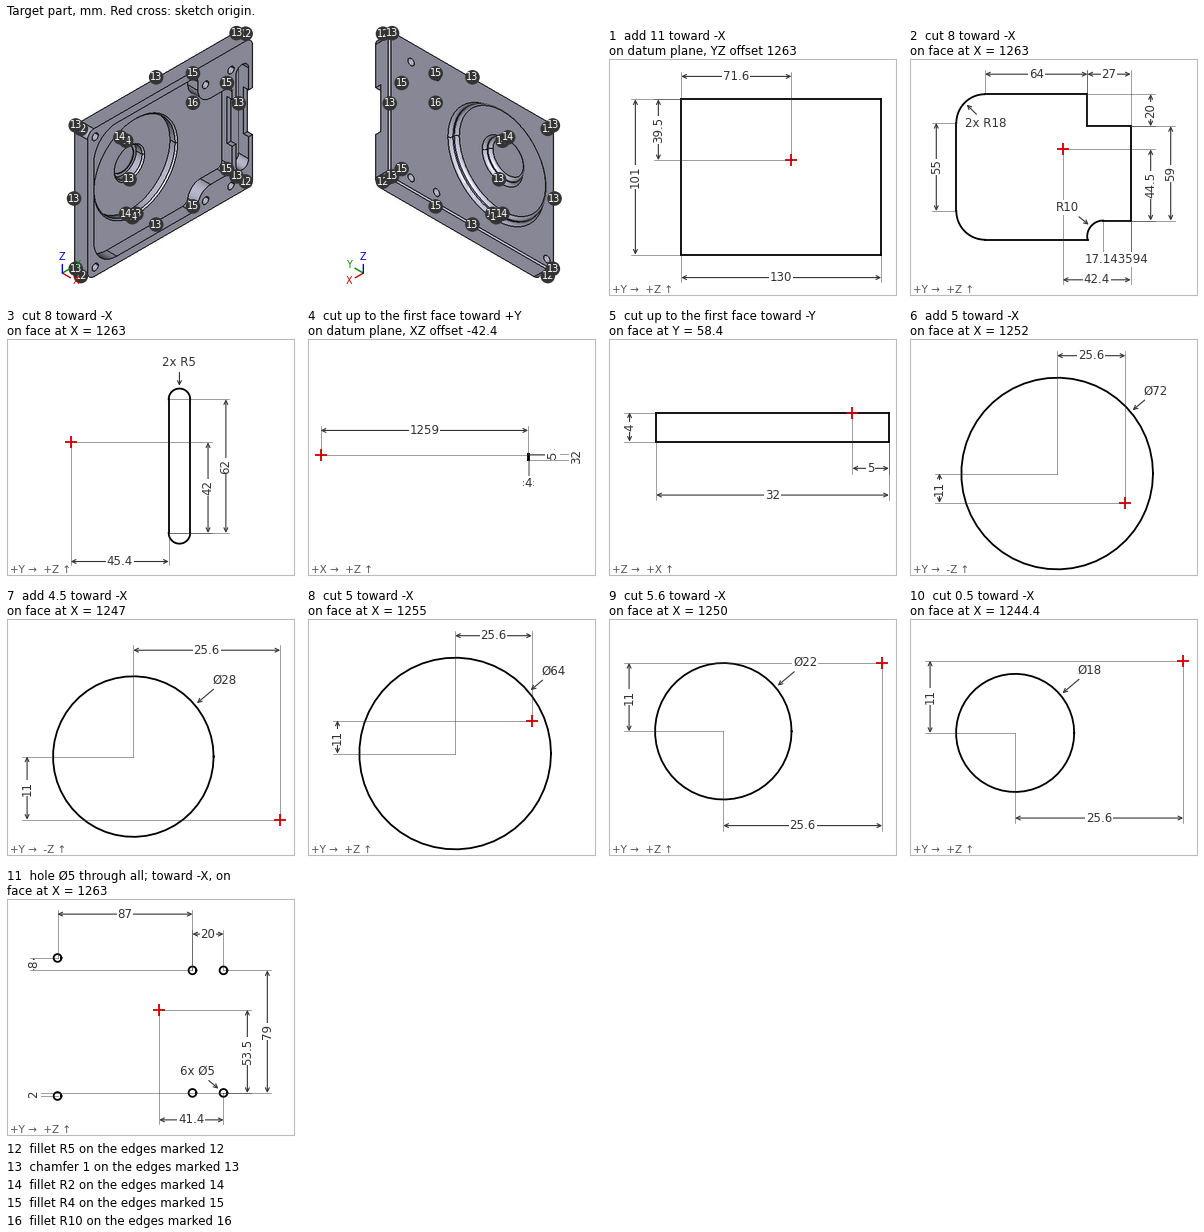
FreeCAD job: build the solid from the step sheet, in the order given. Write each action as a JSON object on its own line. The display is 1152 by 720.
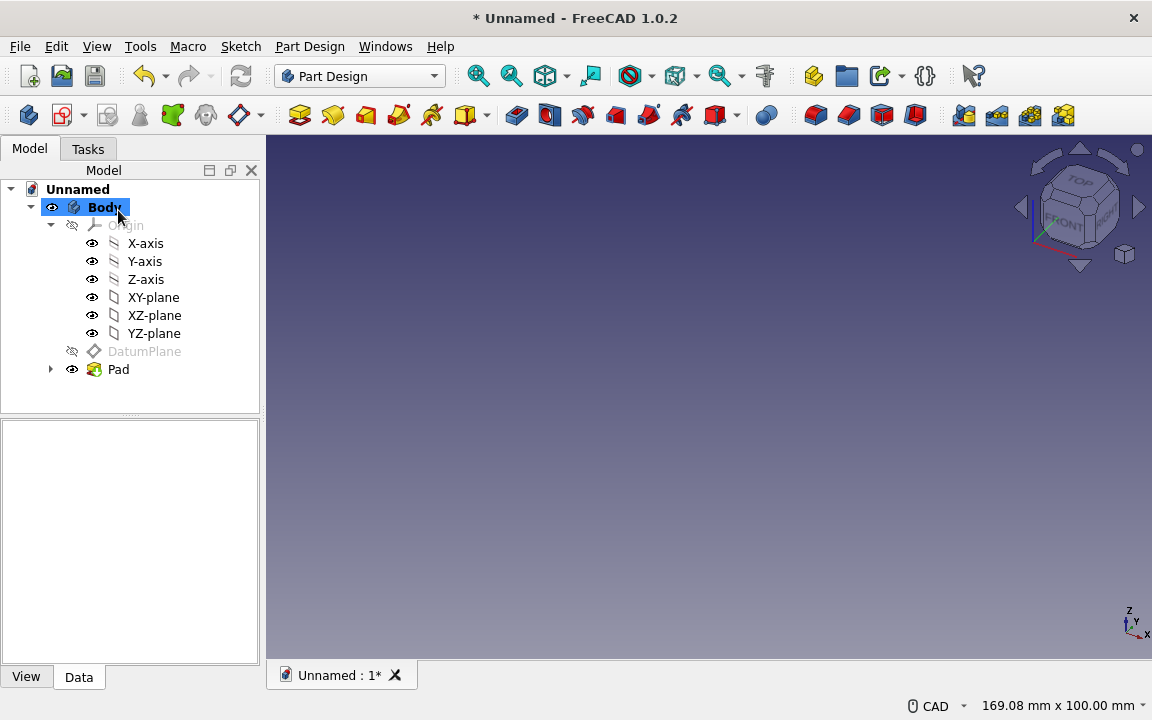
{"action": "left_click", "coordinate": [479, 76]}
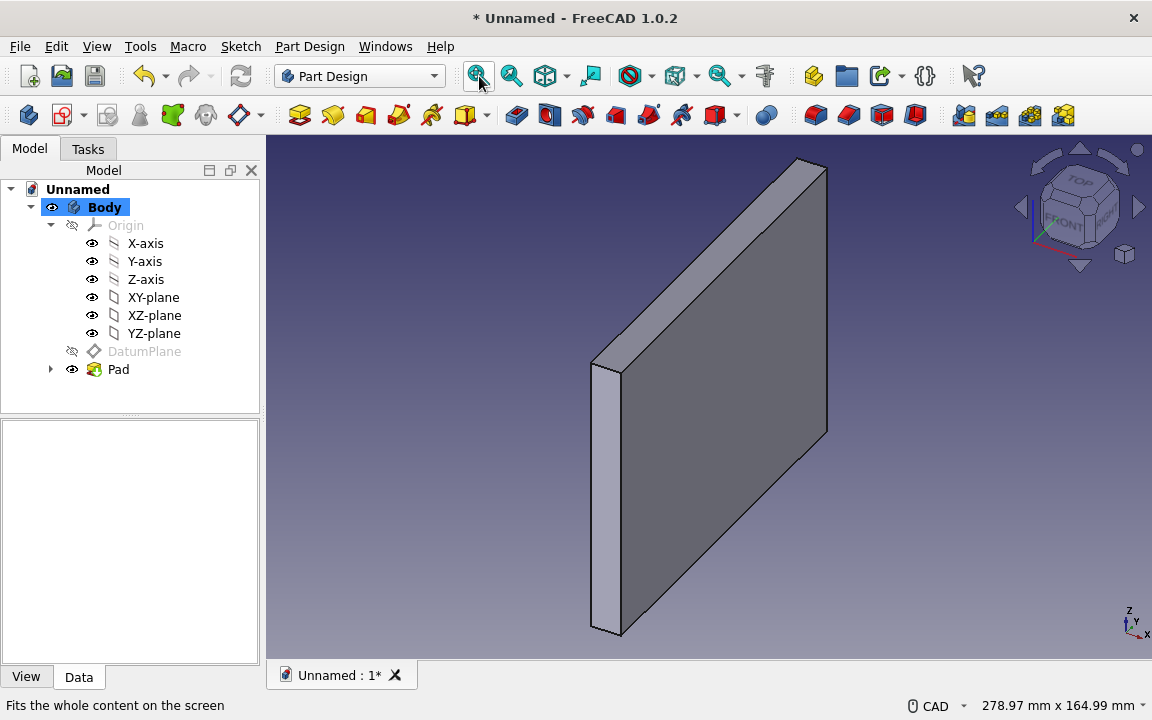
{"action": "left_click", "coordinate": [724, 401]}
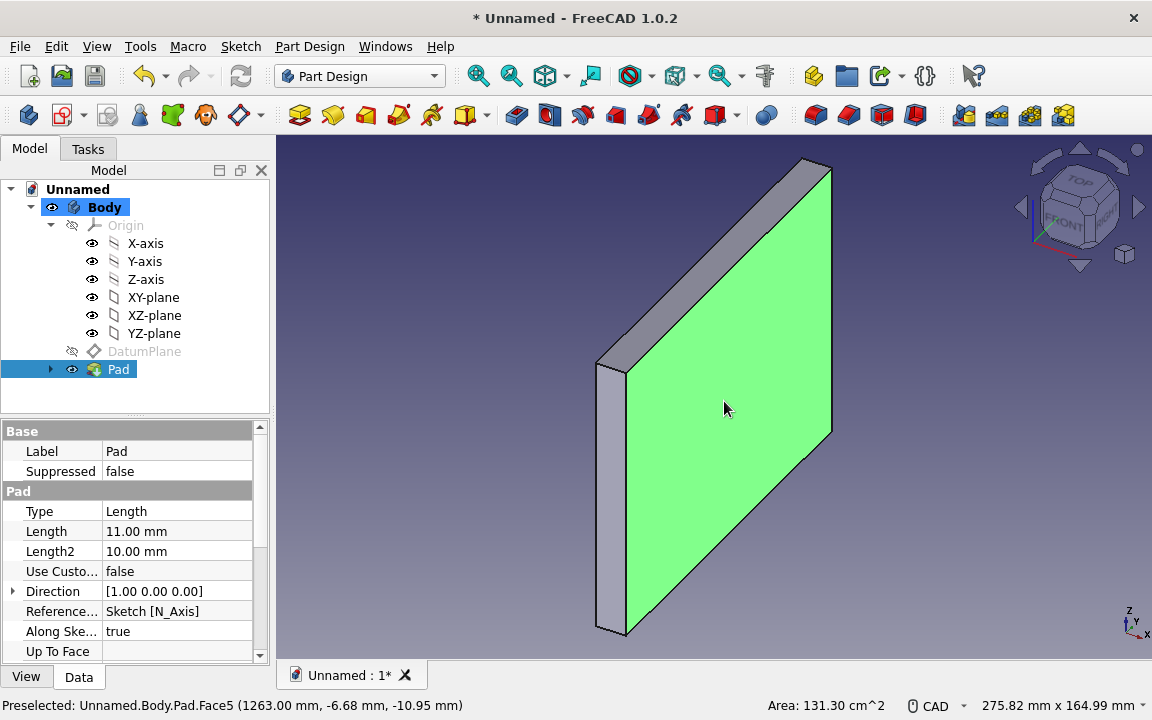
{"action": "left_click", "coordinate": [62, 116]}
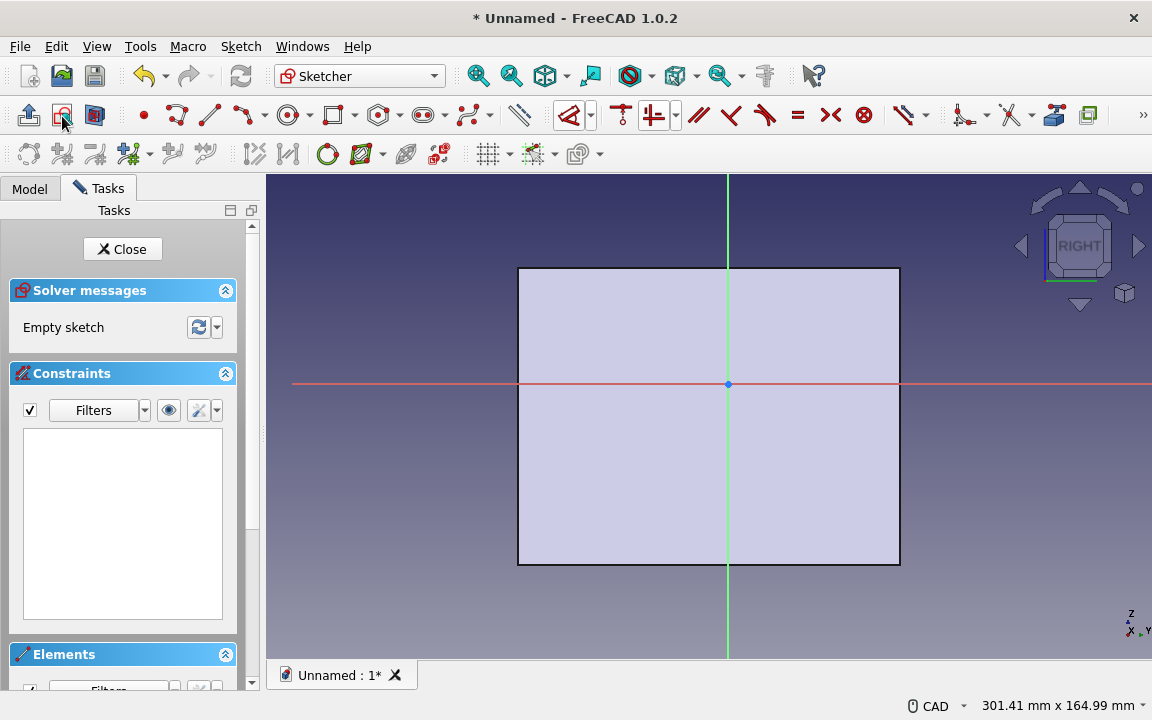
{"action": "left_click", "coordinate": [177, 116]}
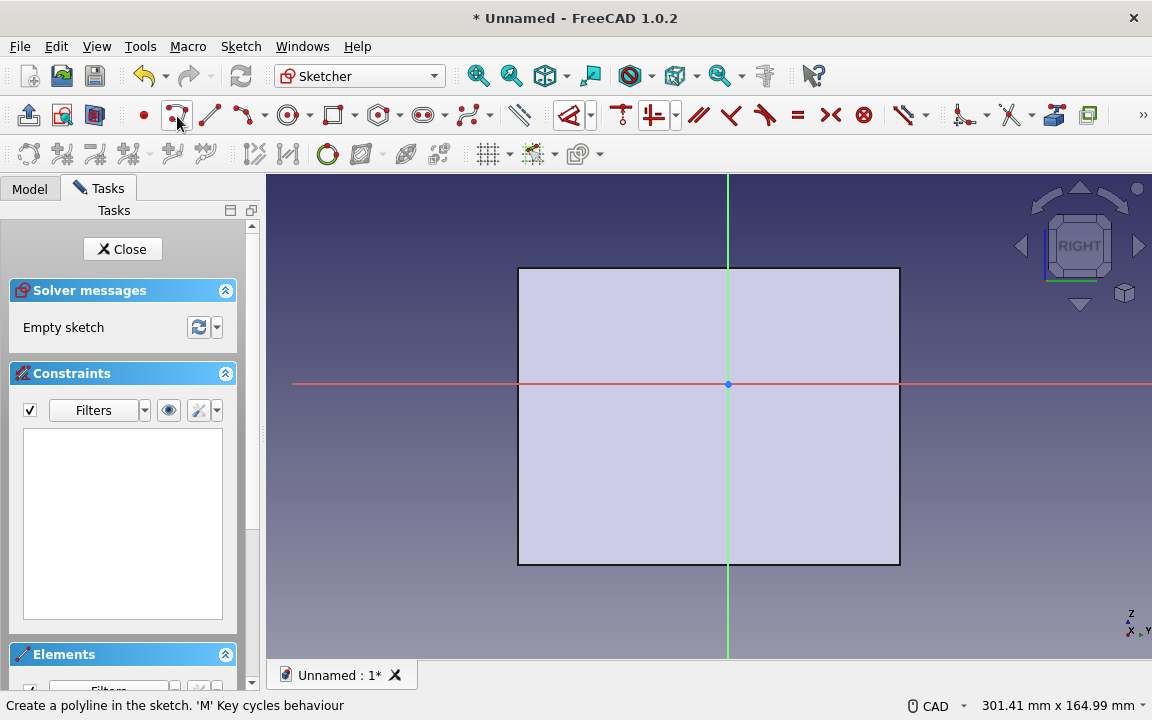
{"action": "left_click", "coordinate": [803, 515]}
{"action": "left_click", "coordinate": [853, 515]}
{"action": "left_click", "coordinate": [853, 342]}
{"action": "left_click", "coordinate": [774, 342]}
{"action": "left_click", "coordinate": [774, 283]}
{"action": "left_click", "coordinate": [586, 283]}
{"action": "right_click", "coordinate": [586, 283]}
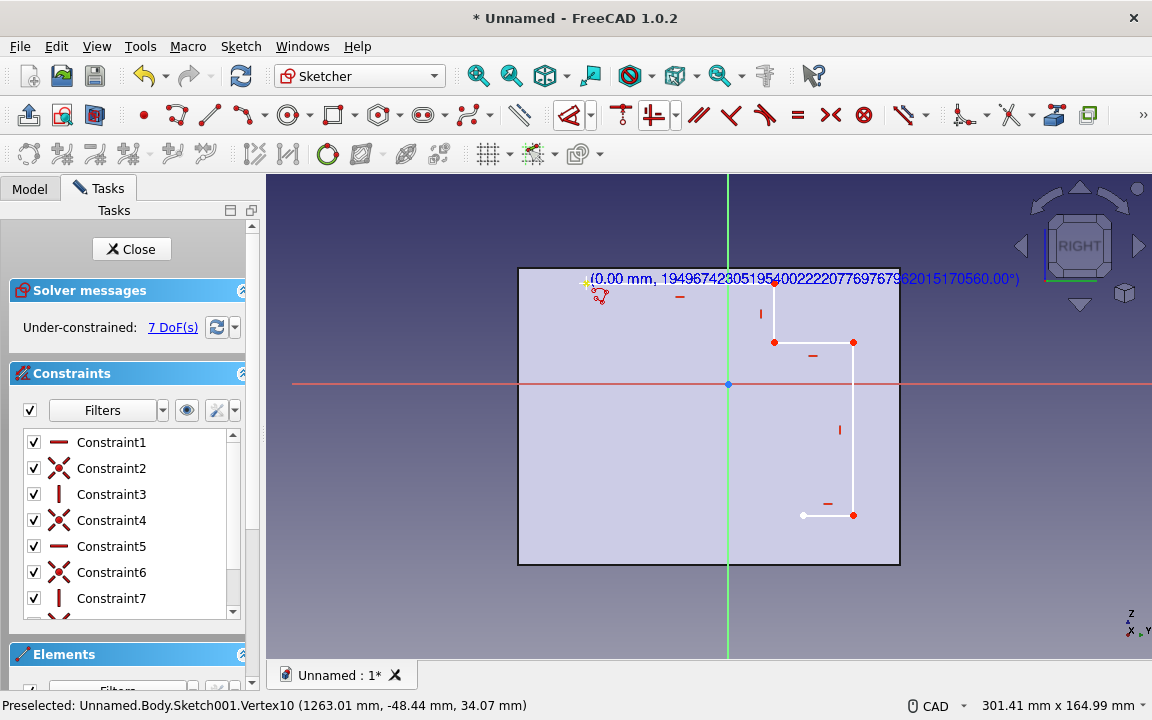
{"action": "left_click", "coordinate": [210, 116]}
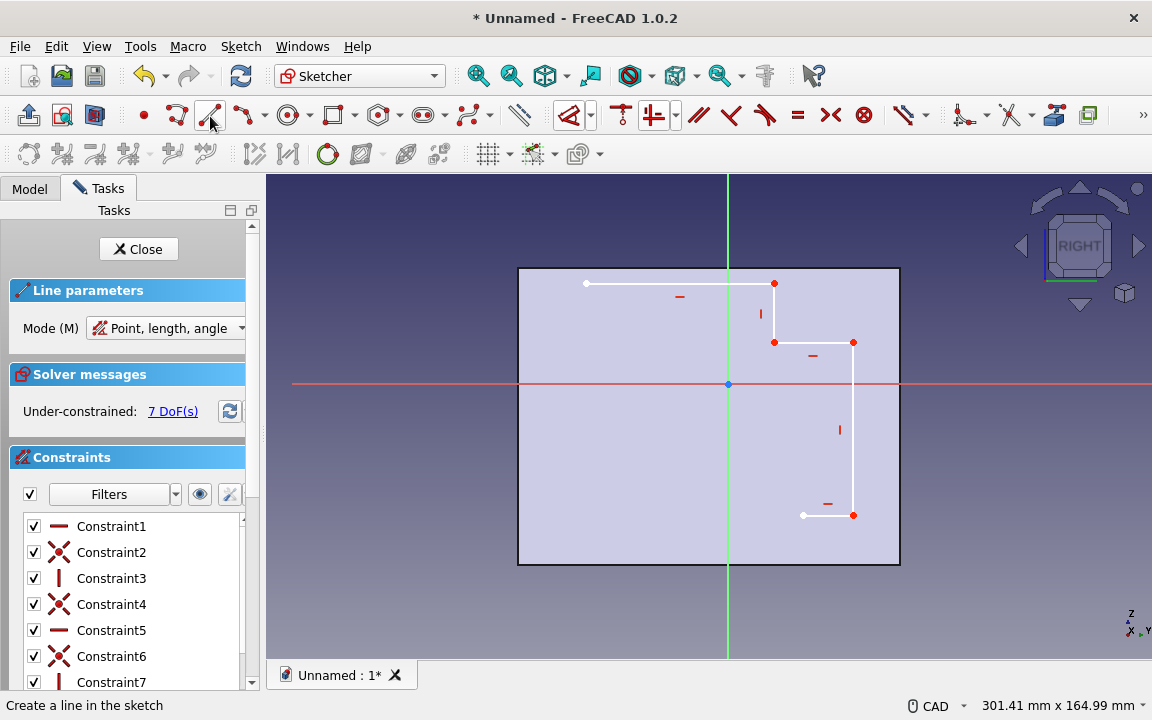
{"action": "left_click", "coordinate": [533, 336]}
{"action": "left_click", "coordinate": [533, 497]}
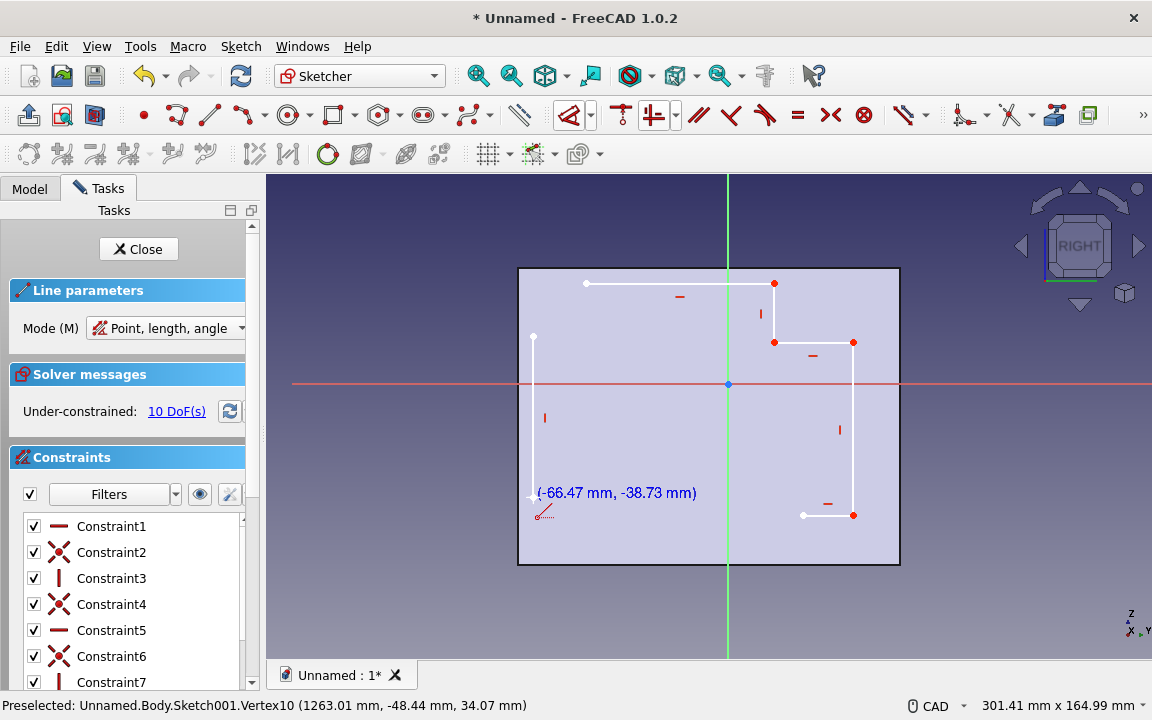
{"action": "left_click", "coordinate": [586, 550]}
{"action": "left_click", "coordinate": [774, 550]}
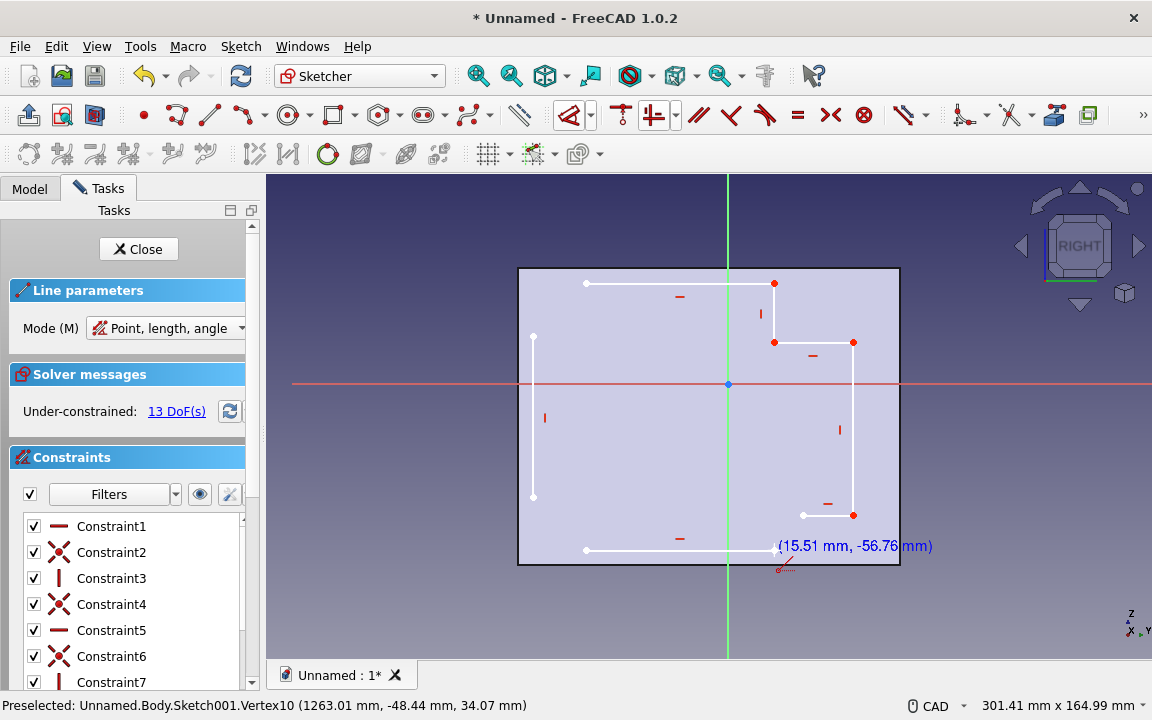
{"action": "left_click", "coordinate": [242, 116]}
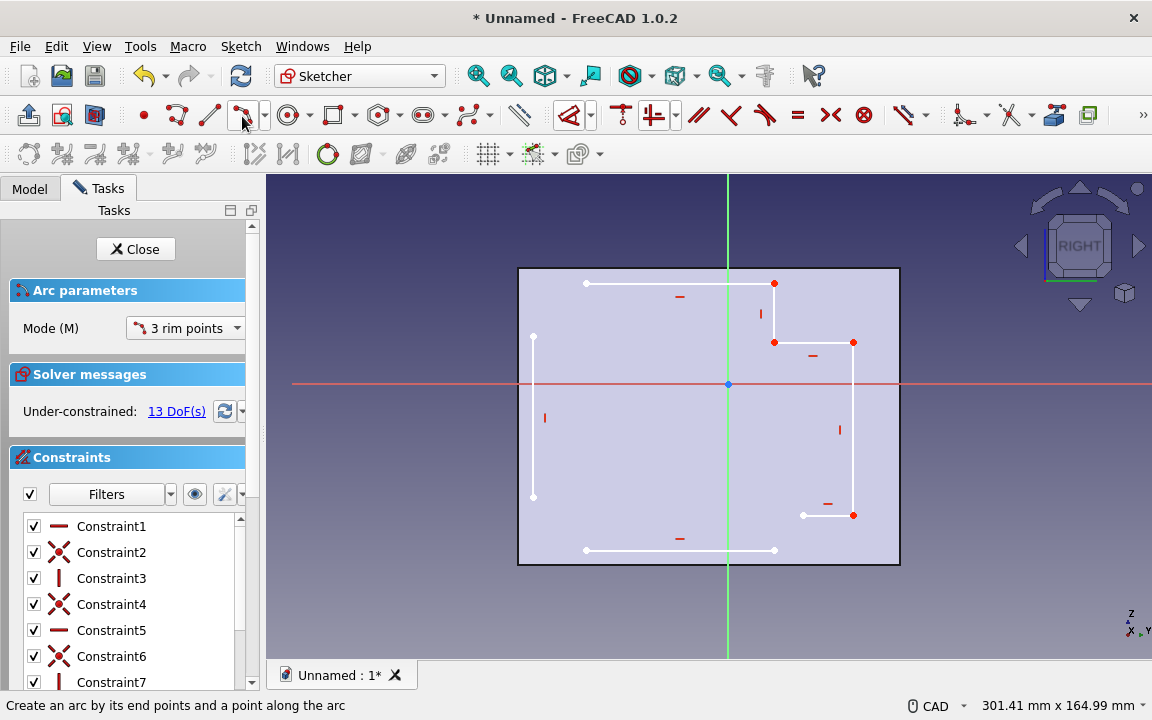
{"action": "left_click", "coordinate": [586, 284]}
{"action": "left_click", "coordinate": [533, 337]}
{"action": "left_click", "coordinate": [548, 298]}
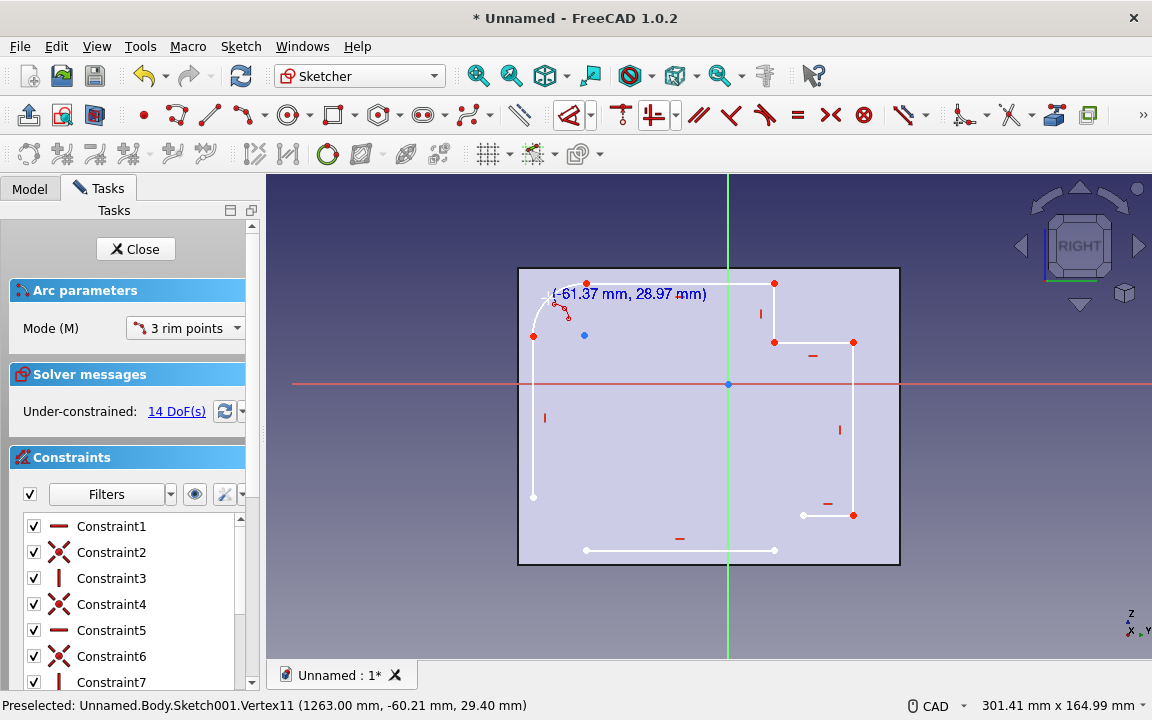
{"action": "left_click", "coordinate": [533, 498]}
{"action": "left_click", "coordinate": [586, 551]}
{"action": "left_click", "coordinate": [548, 535]}